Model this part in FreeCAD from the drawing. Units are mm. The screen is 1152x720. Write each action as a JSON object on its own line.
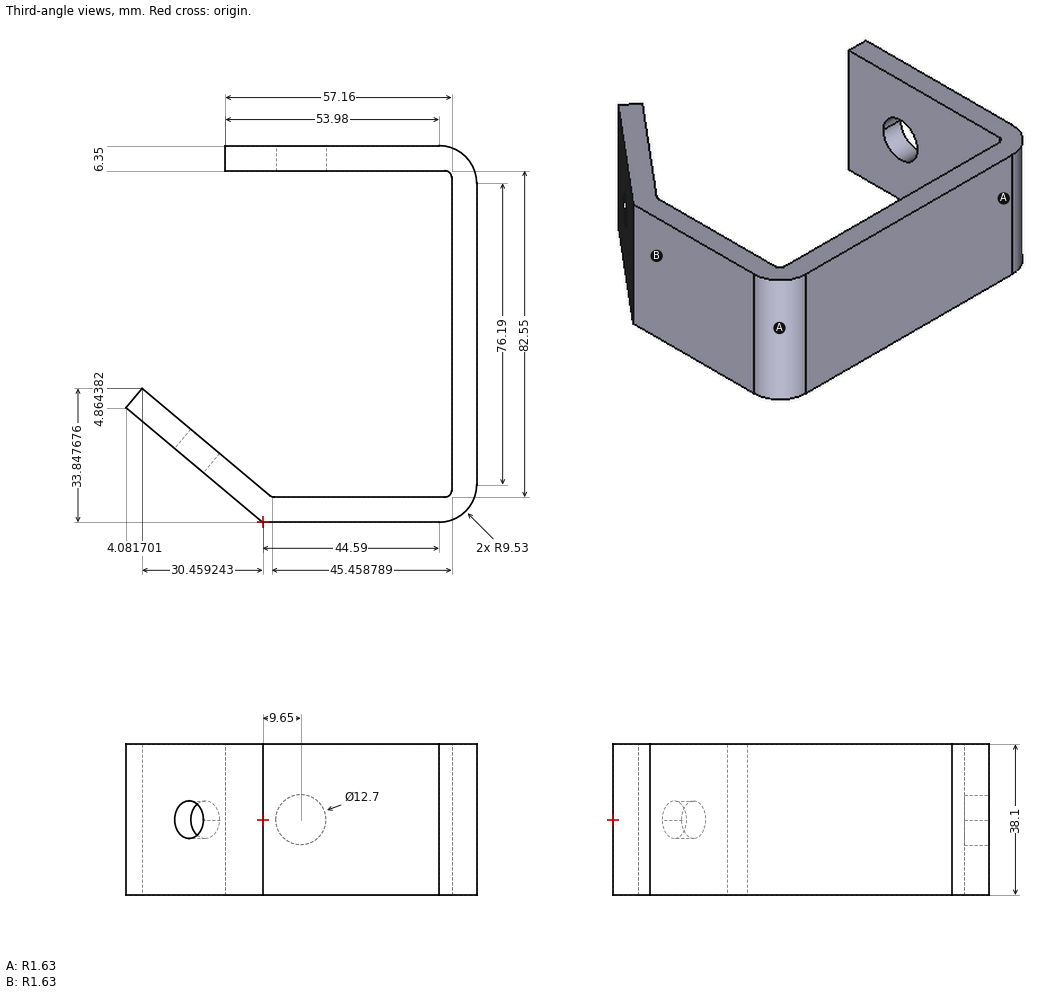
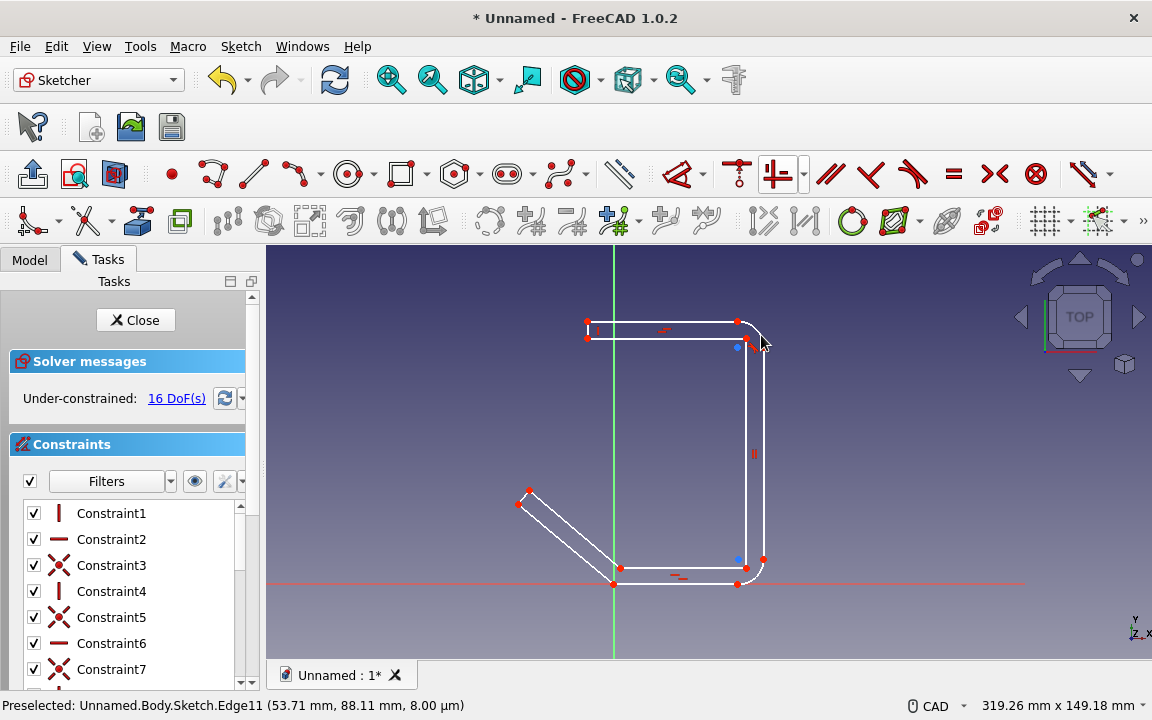
{"action": "left_click", "coordinate": [764, 496]}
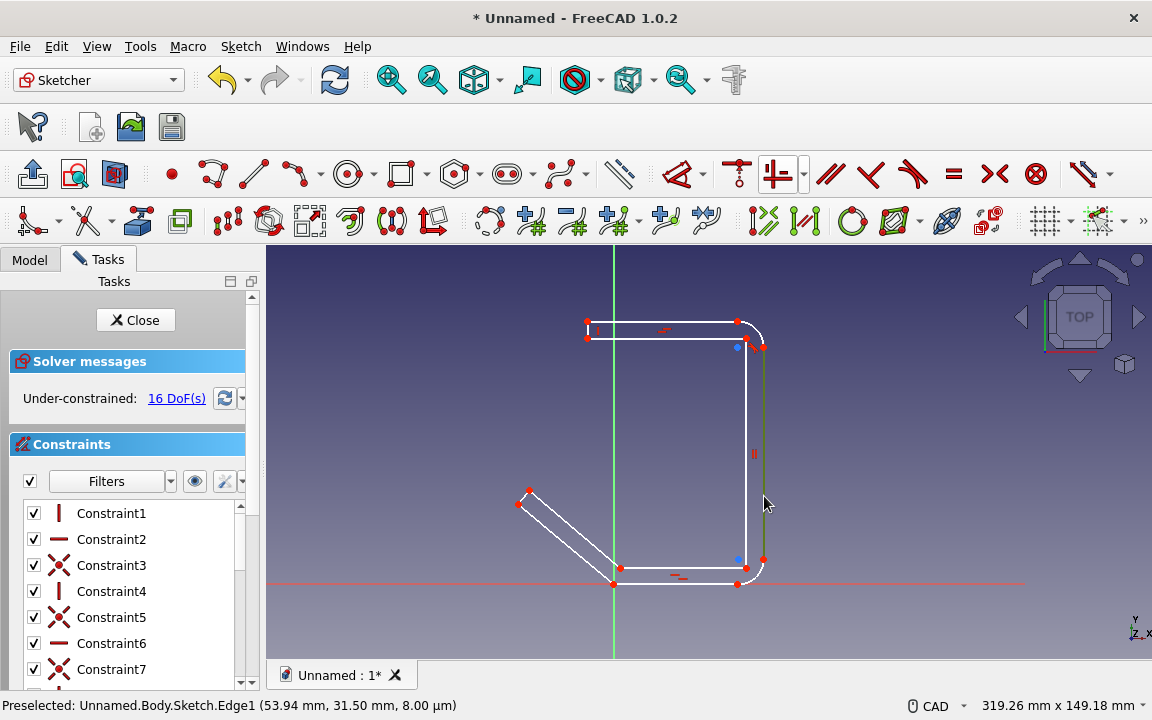
{"action": "left_click", "coordinate": [749, 582]}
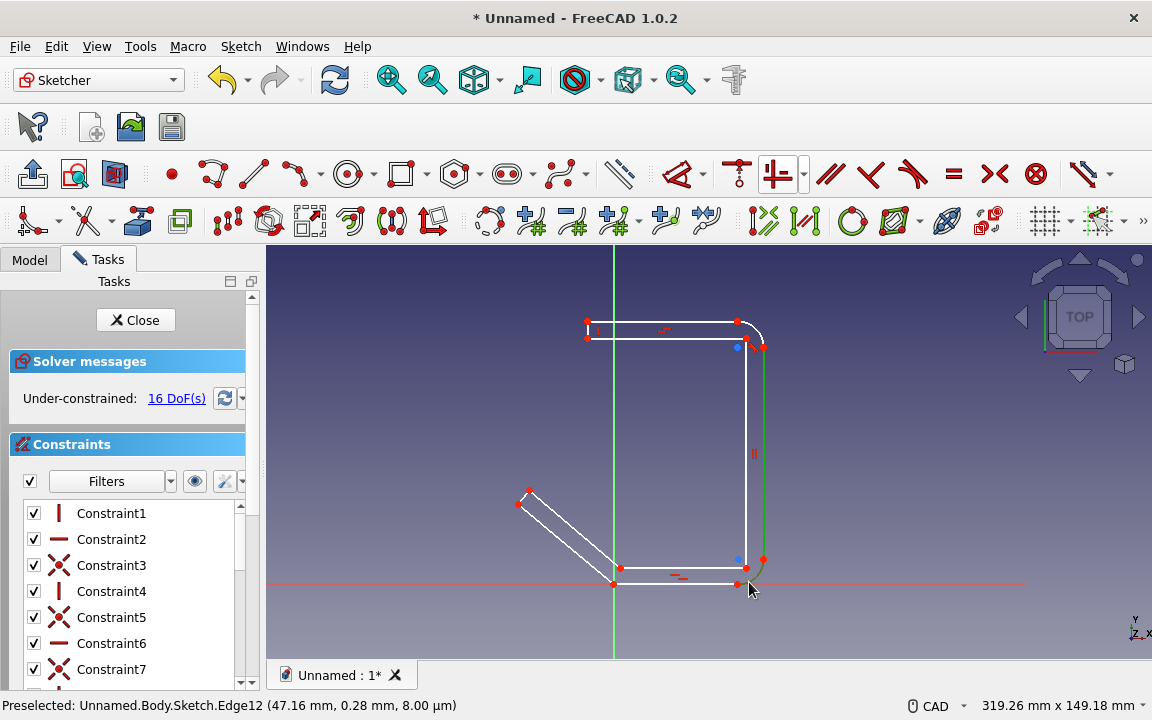
{"action": "key", "text": "t"}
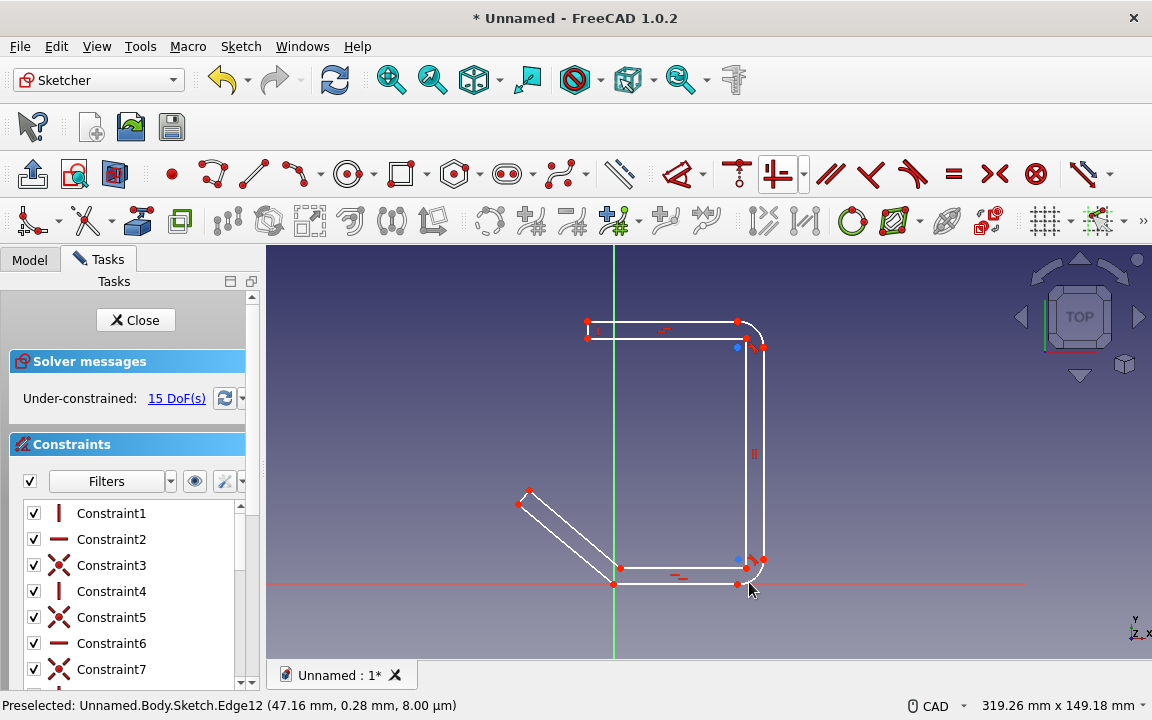
{"action": "left_click", "coordinate": [693, 322]}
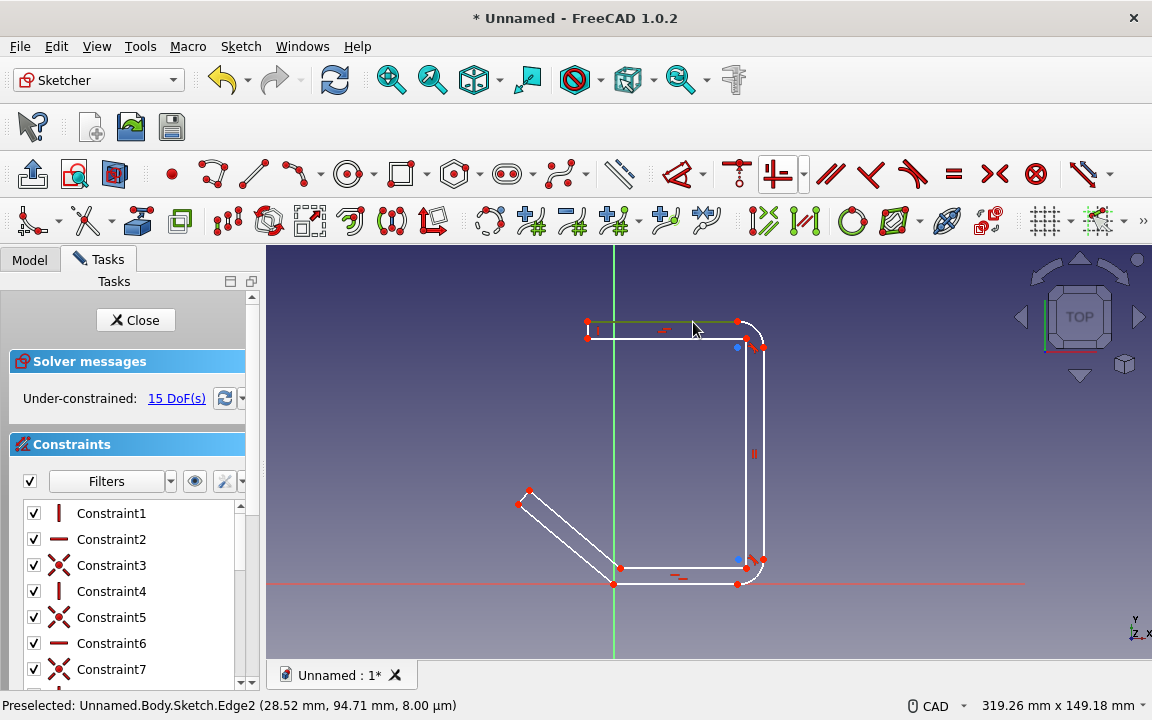
{"action": "left_click", "coordinate": [761, 336]}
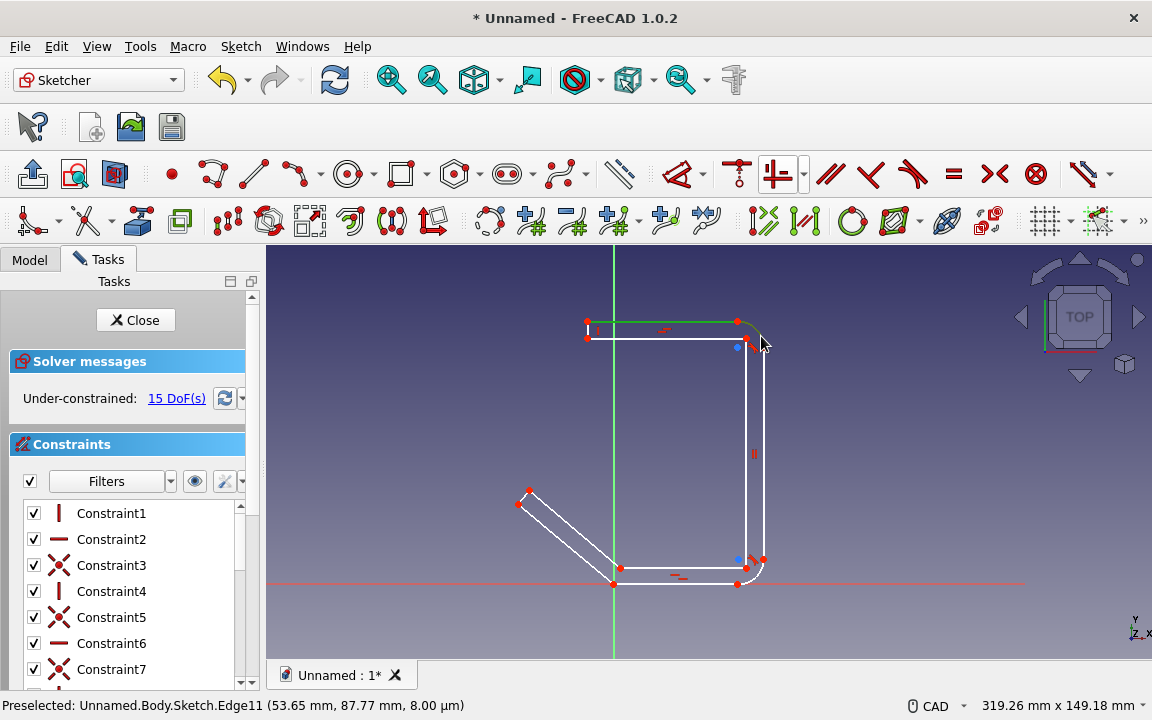
{"action": "left_click", "coordinate": [913, 174]}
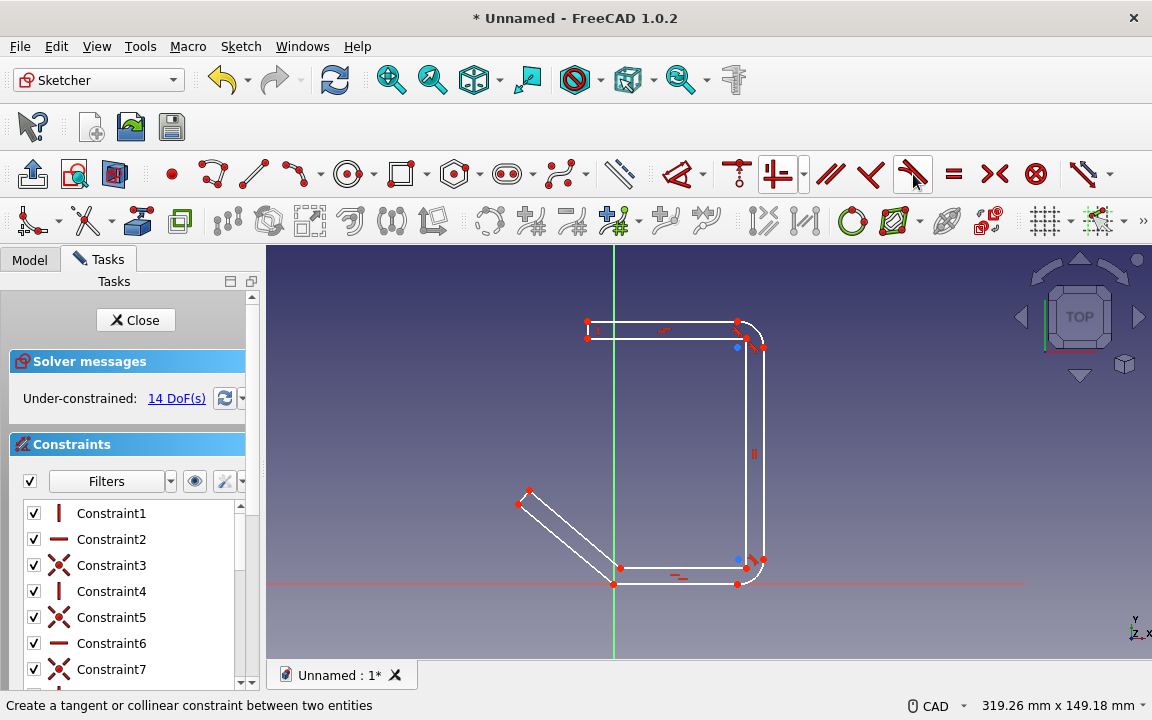
{"action": "left_click", "coordinate": [651, 584]}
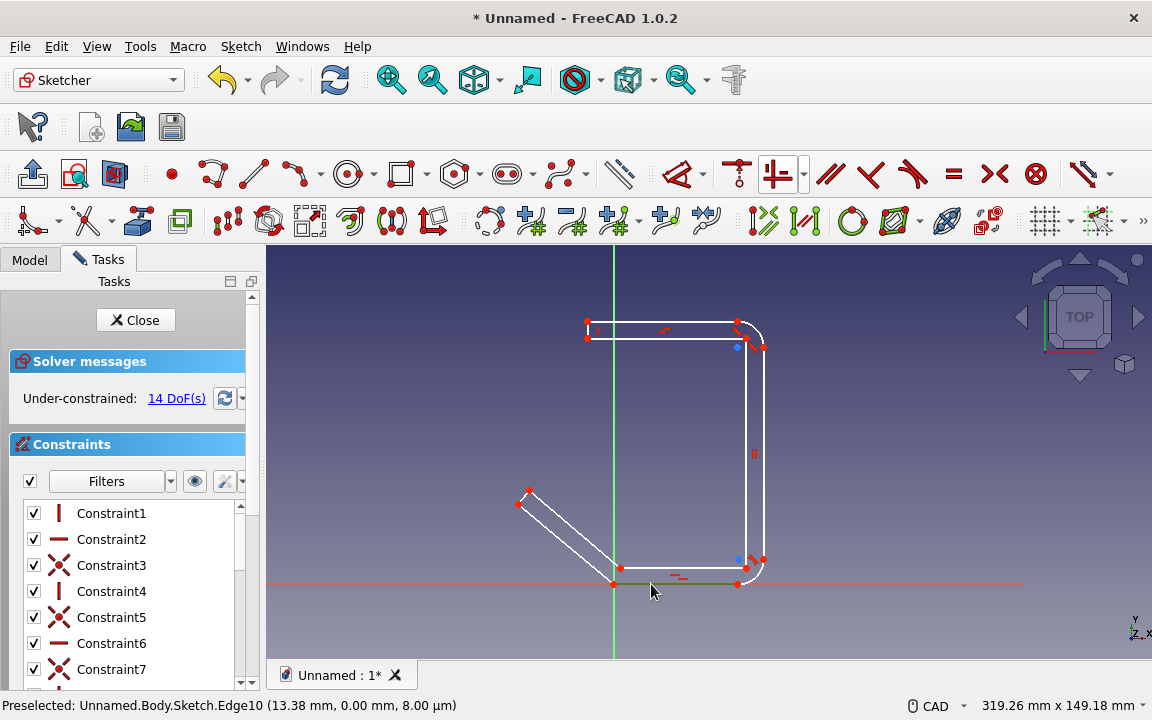
{"action": "left_click", "coordinate": [749, 582]}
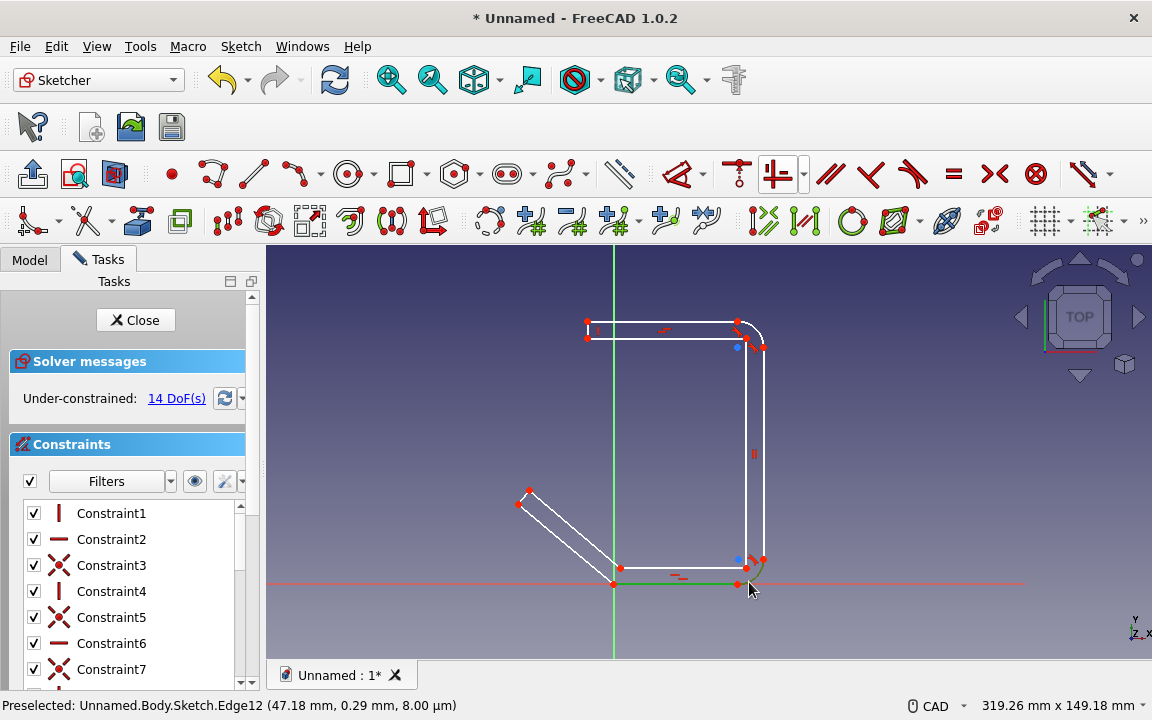
{"action": "key", "text": "t"}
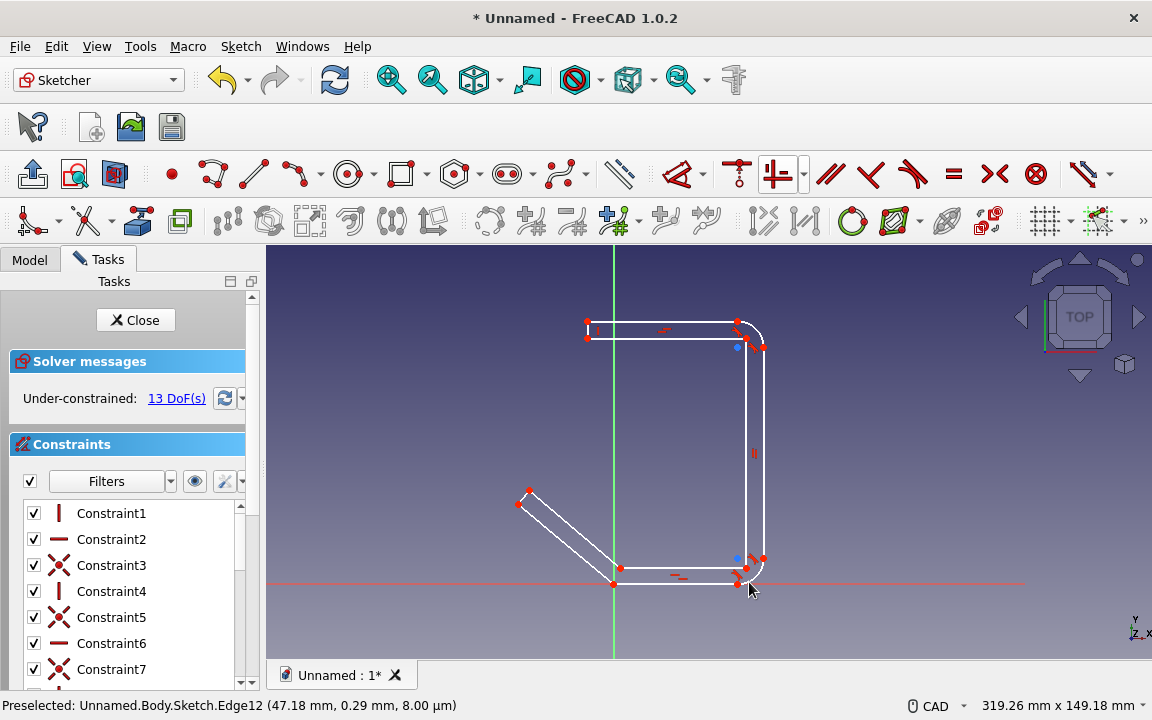
{"action": "left_click", "coordinate": [761, 336]}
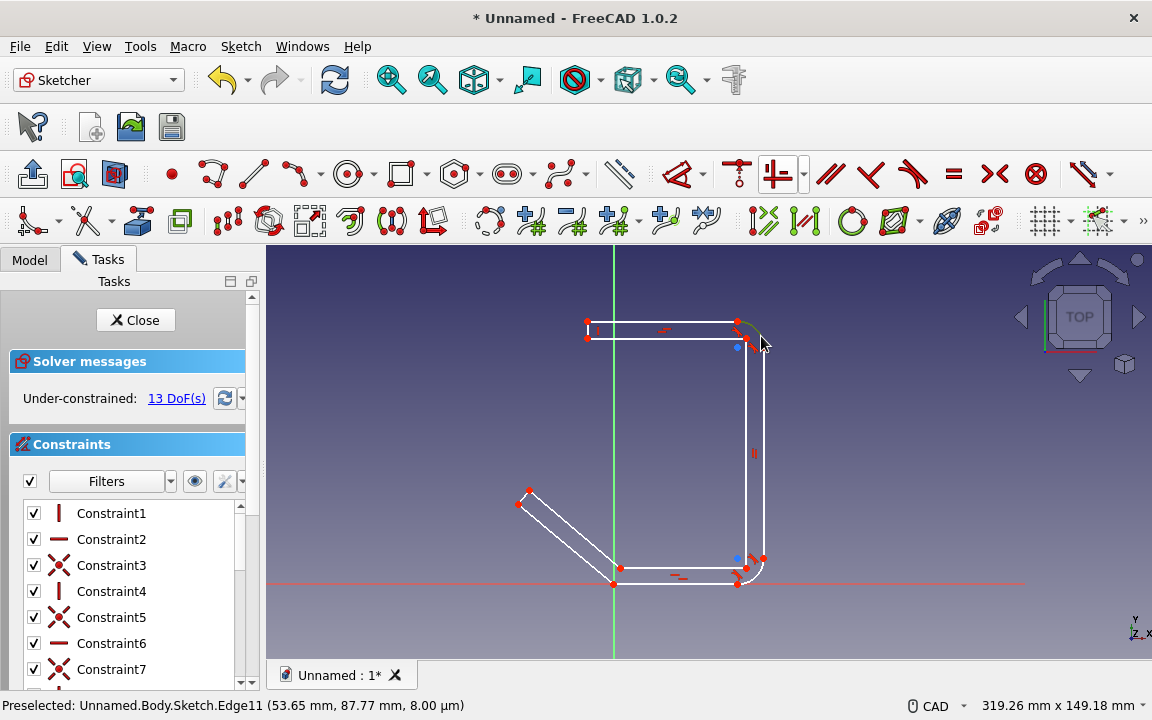
{"action": "left_click", "coordinate": [749, 582]}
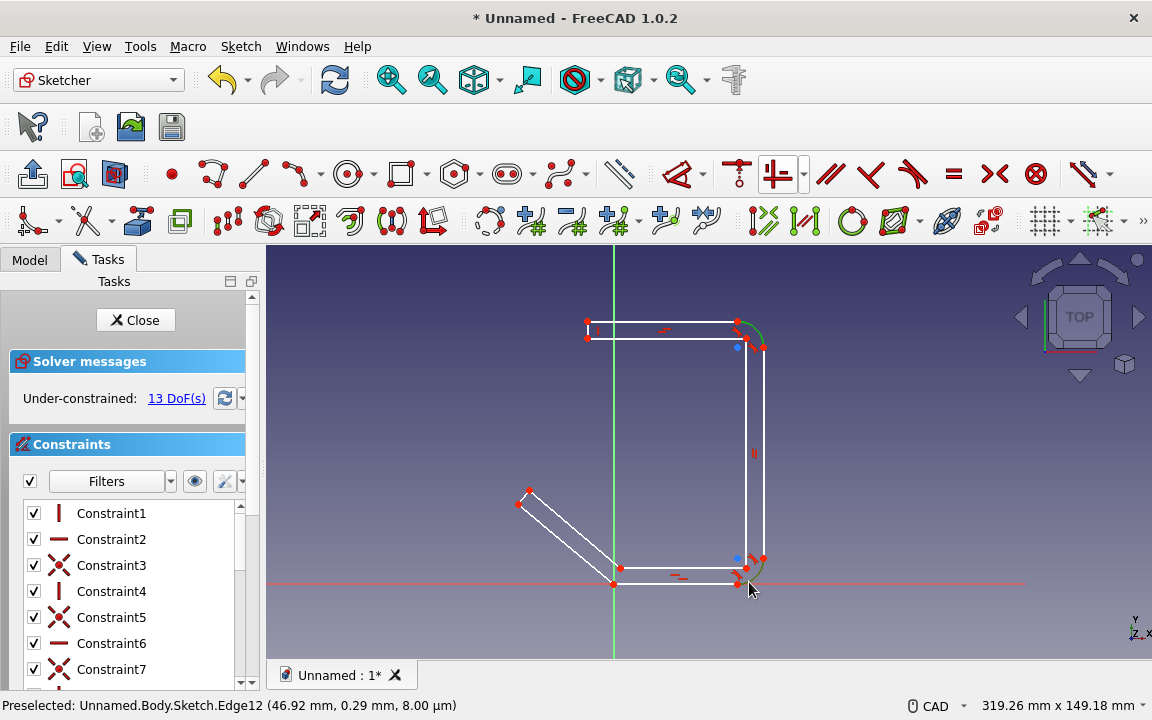
{"action": "left_click", "coordinate": [954, 174]}